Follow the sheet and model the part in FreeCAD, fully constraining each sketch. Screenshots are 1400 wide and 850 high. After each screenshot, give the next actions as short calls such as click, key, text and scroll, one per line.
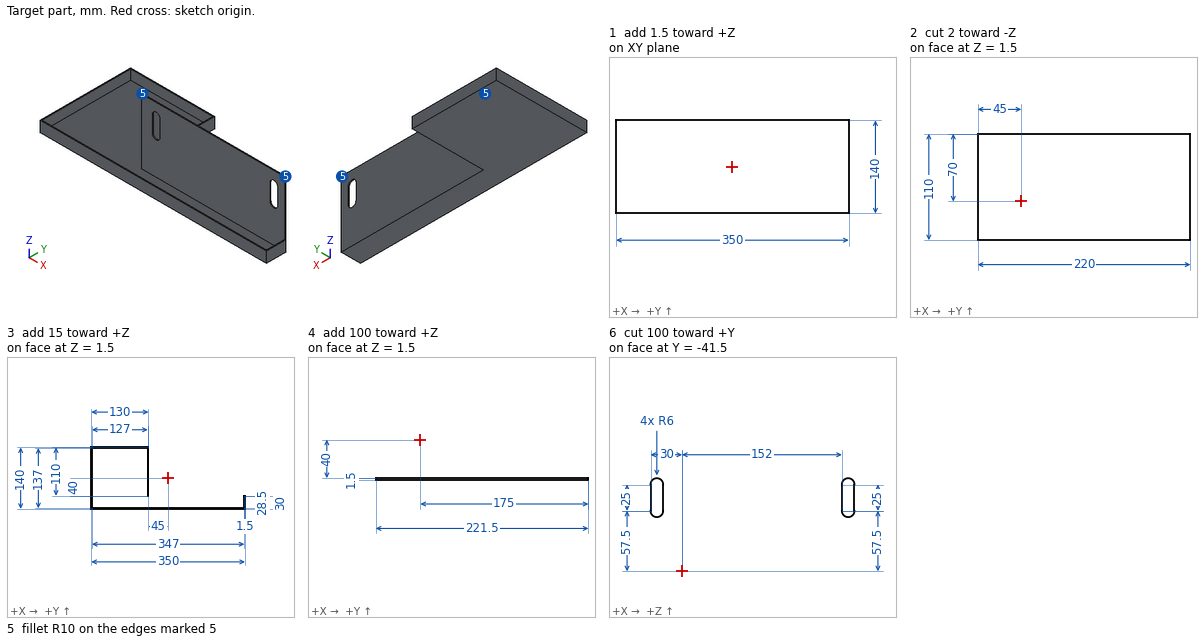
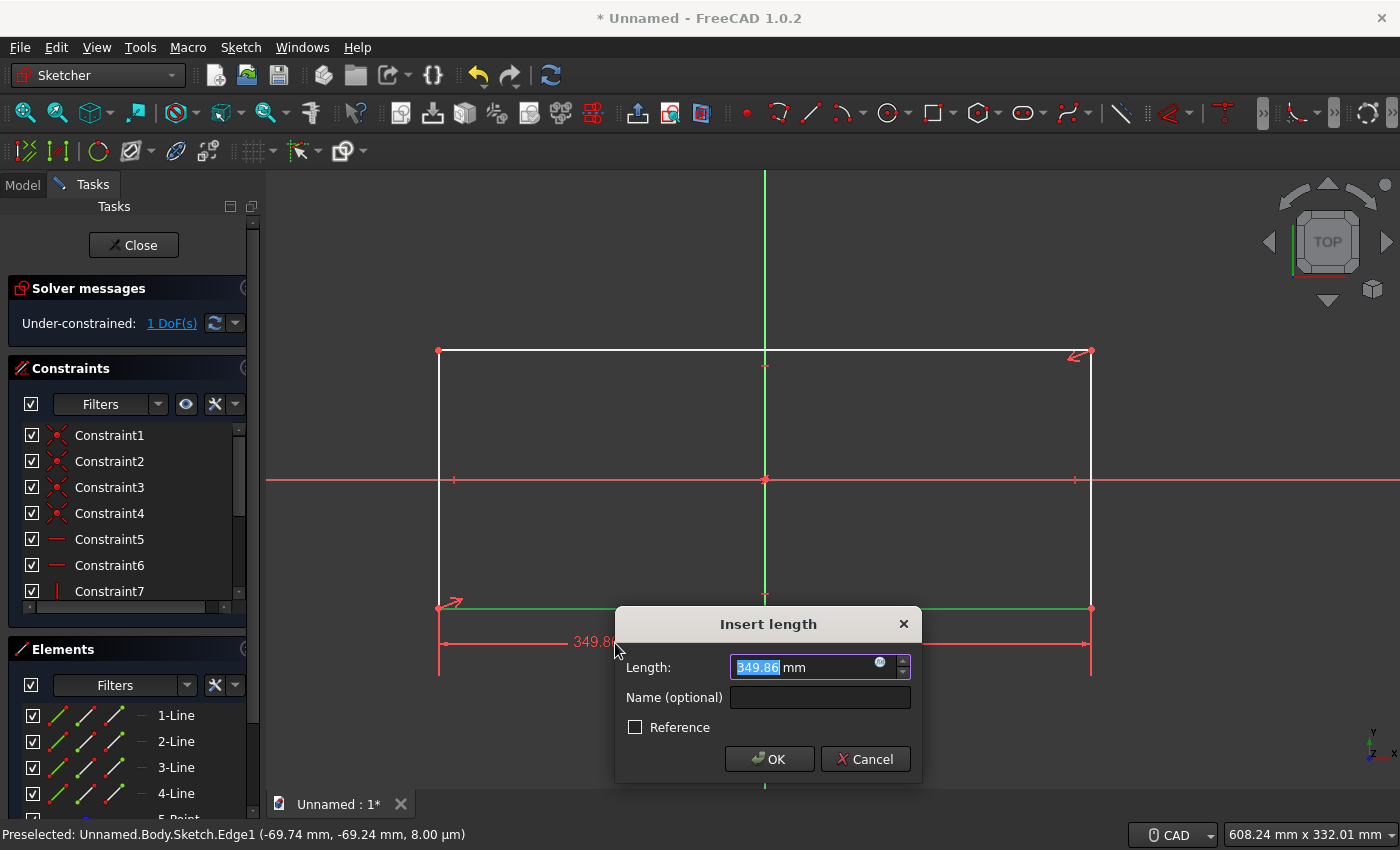
text(350)
key(Return)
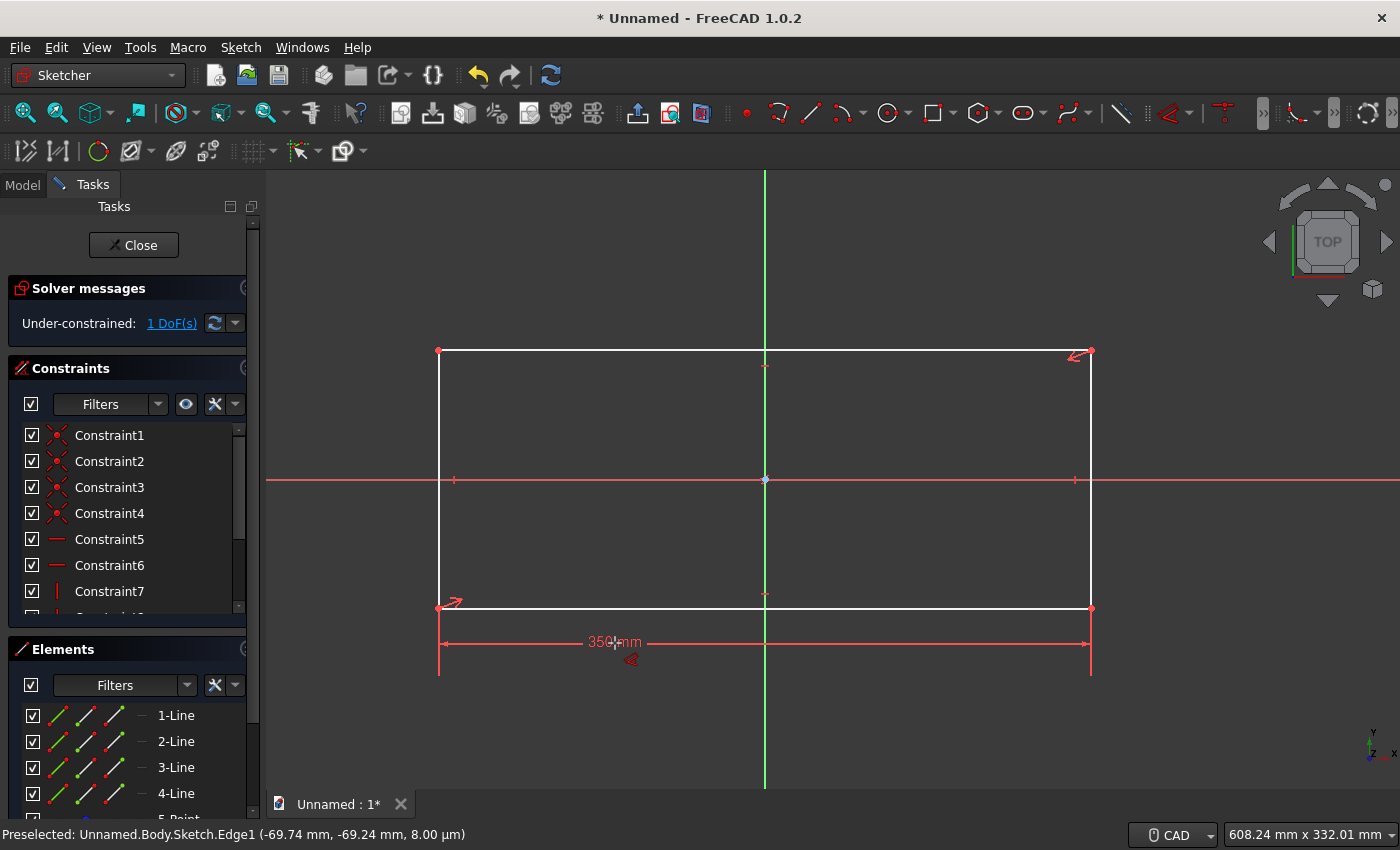
click(1091, 531)
click(1125, 420)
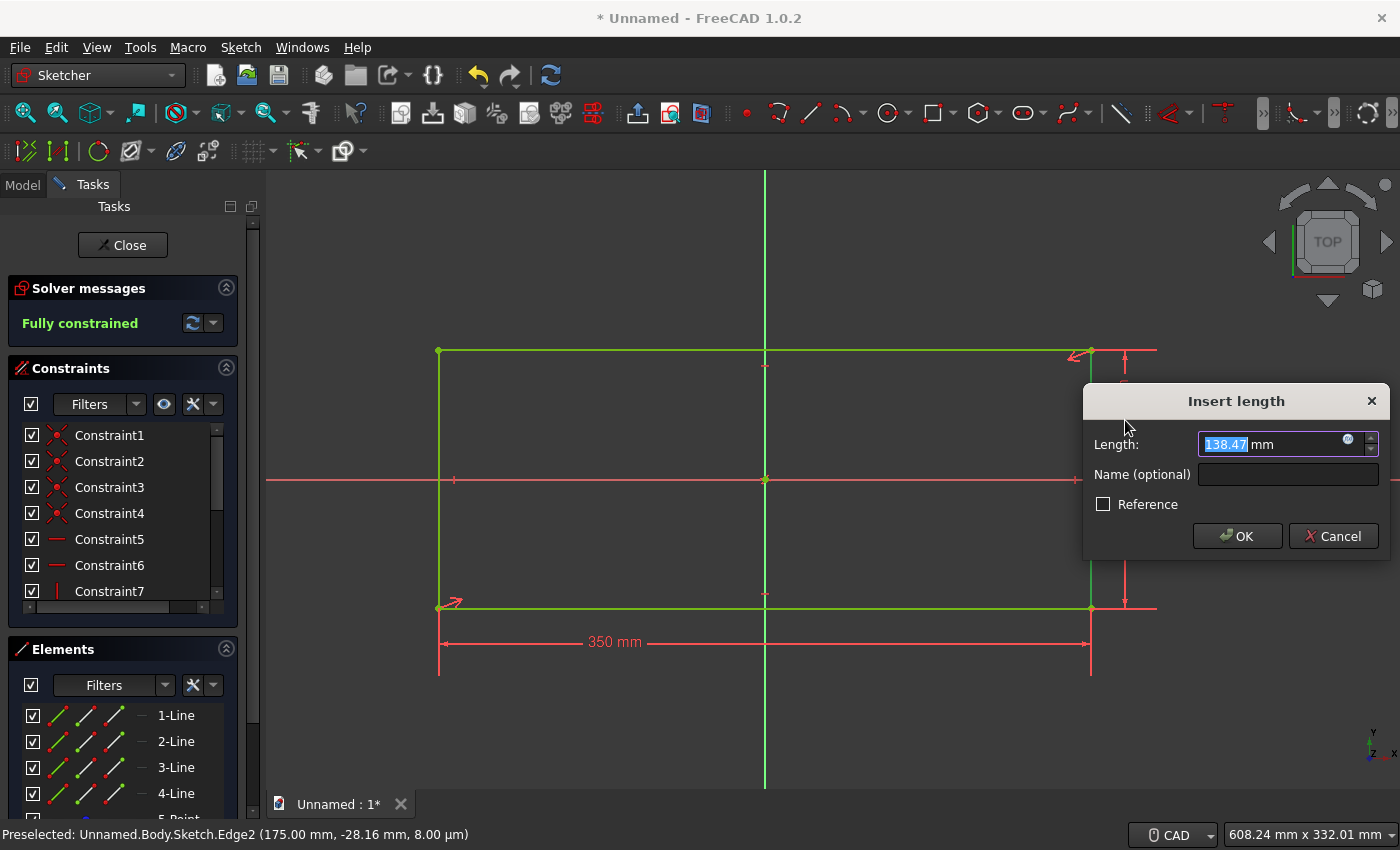
text(140)
key(Return)
key(Escape)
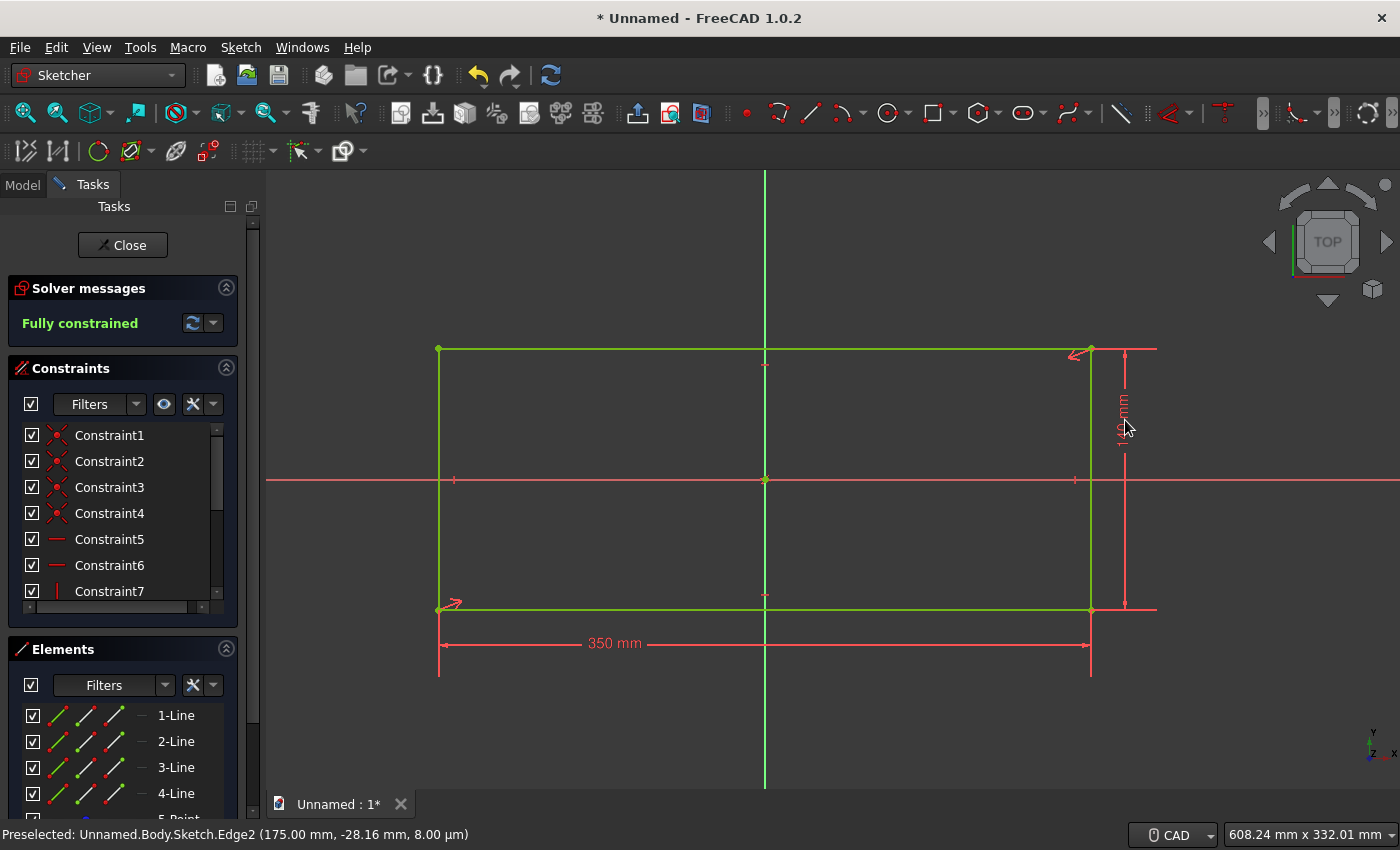
click(123, 245)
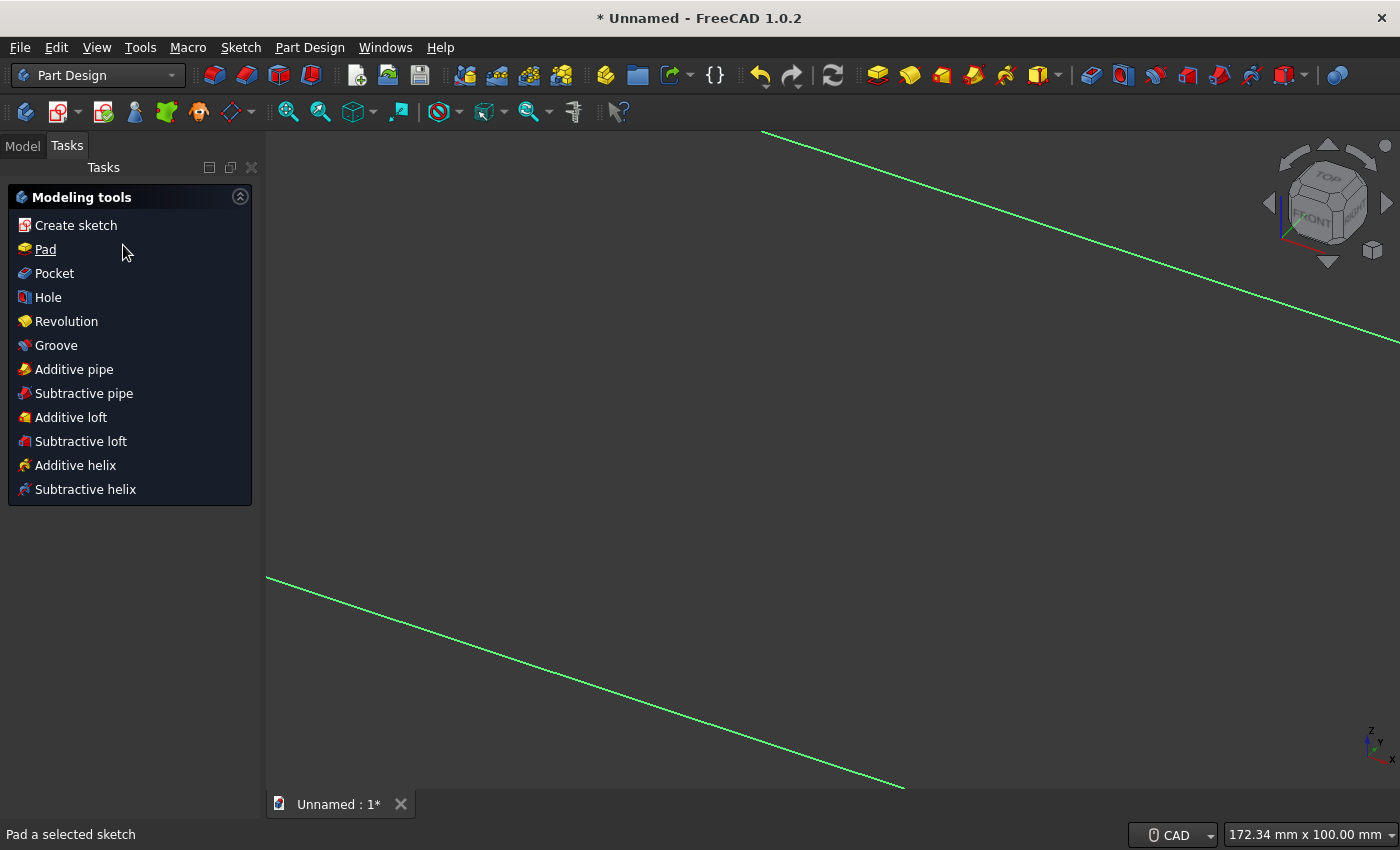
click(878, 76)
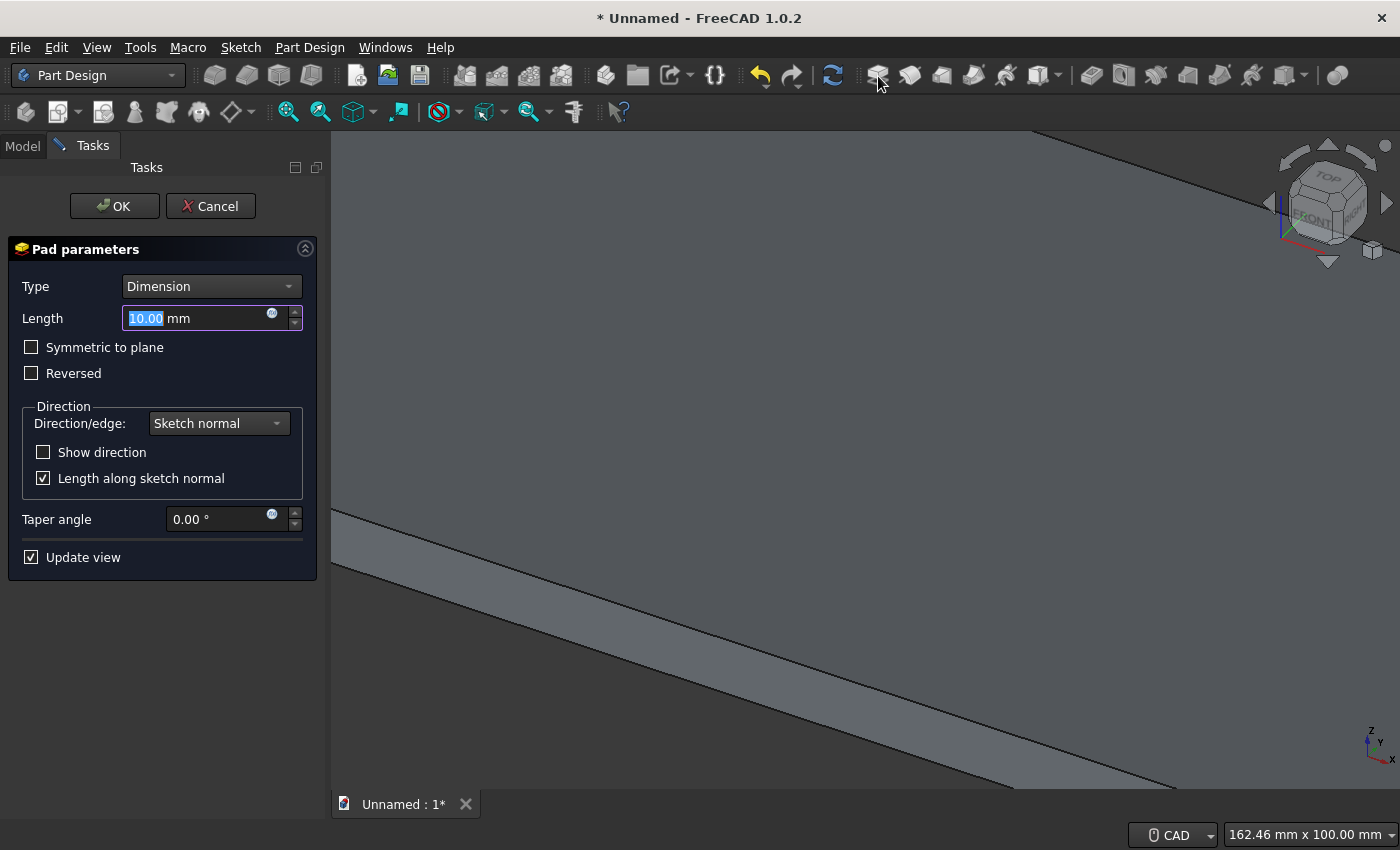
text(1.5)
key(Tab)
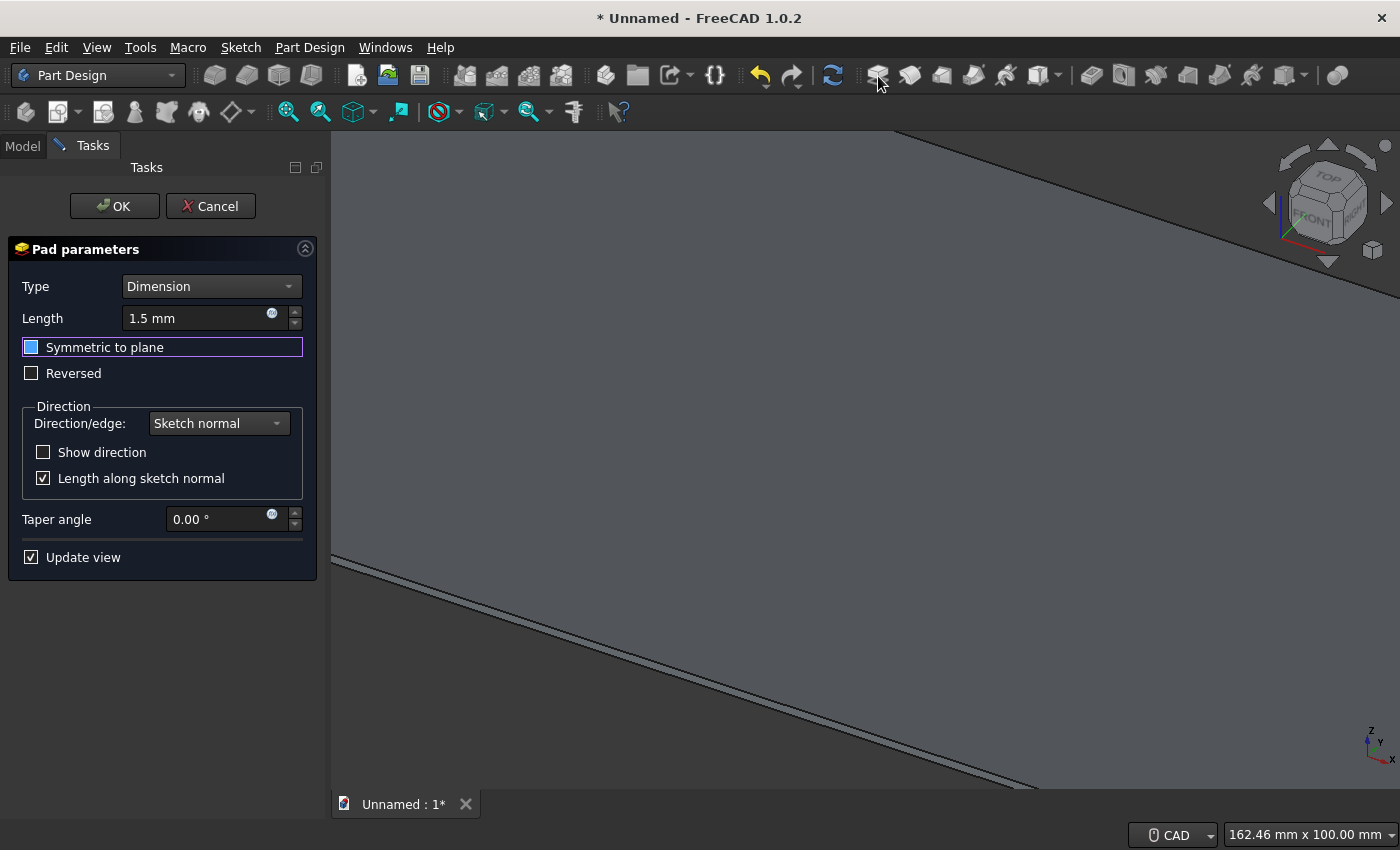
click(115, 206)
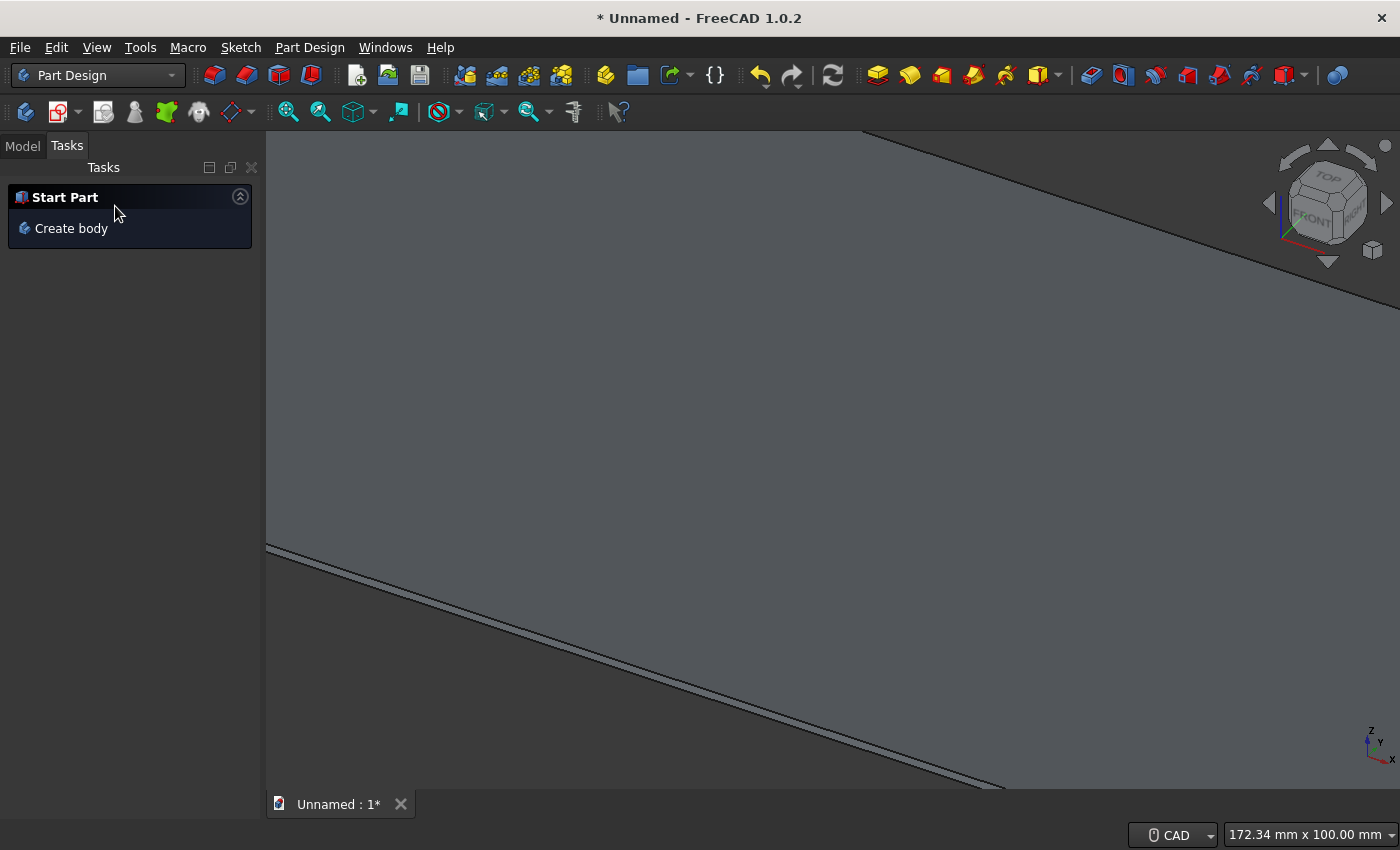
click(290, 112)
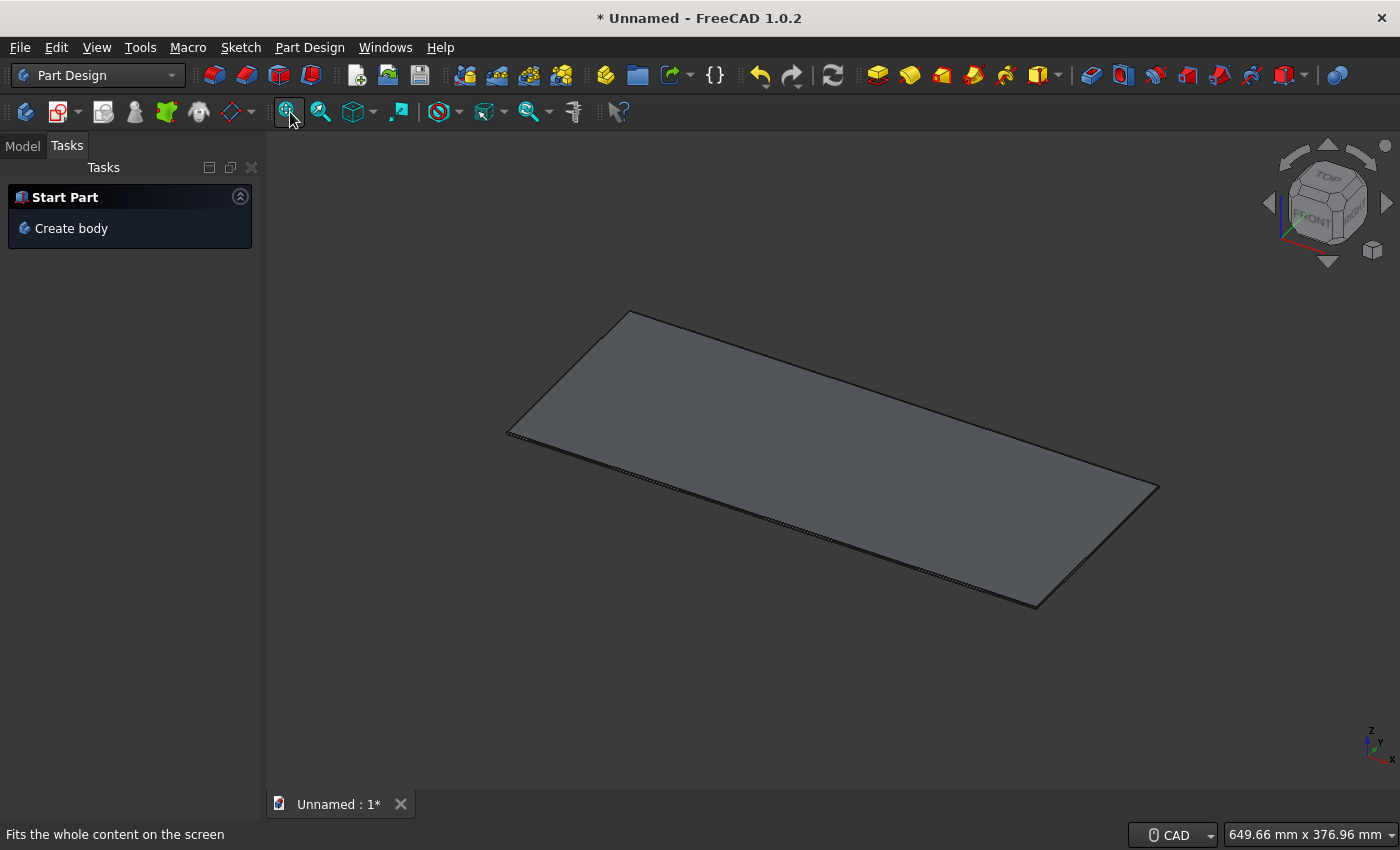
click(984, 508)